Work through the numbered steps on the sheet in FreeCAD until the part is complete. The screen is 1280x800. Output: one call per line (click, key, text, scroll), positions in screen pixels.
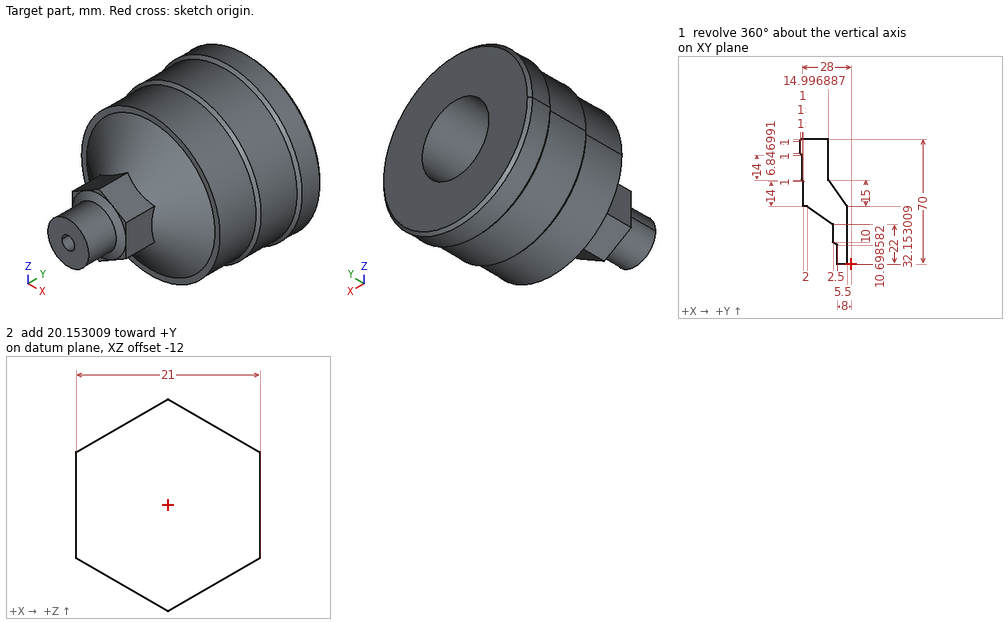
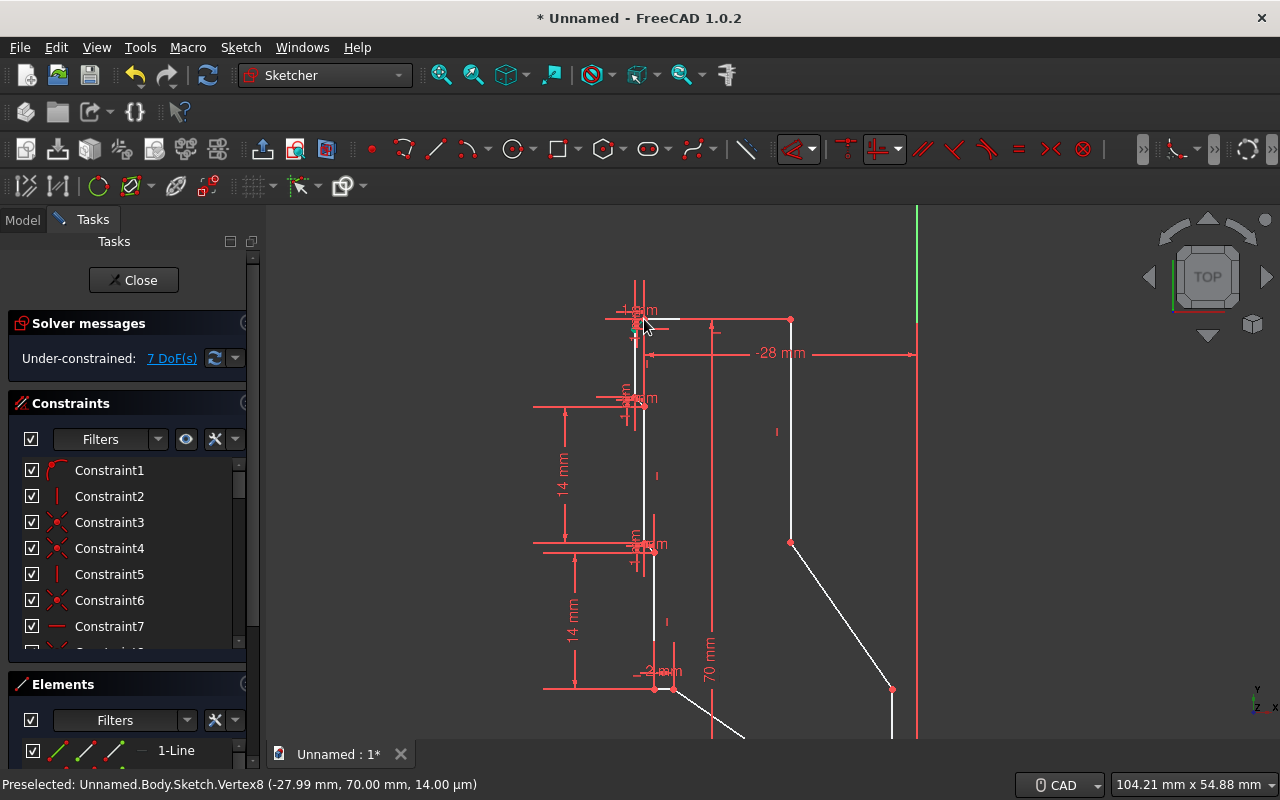
scroll(646, 319, down, 4)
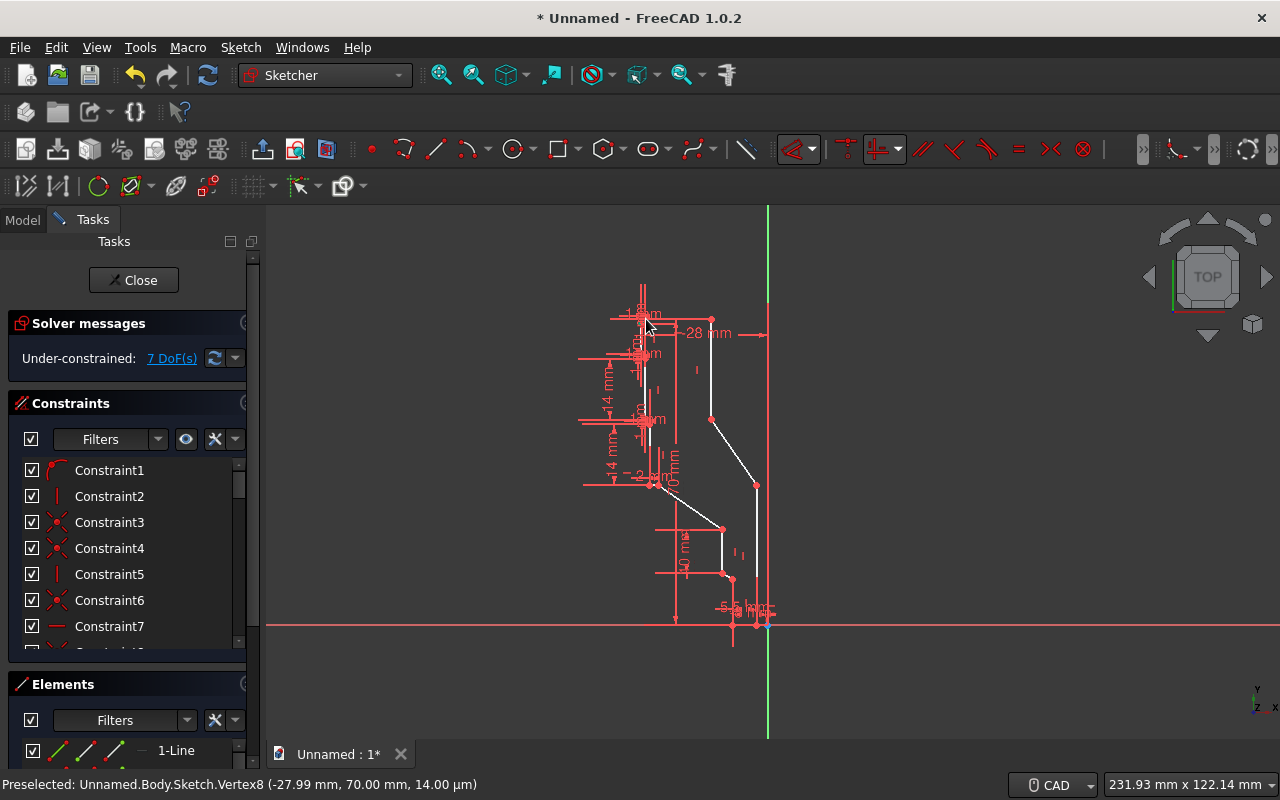
click(722, 530)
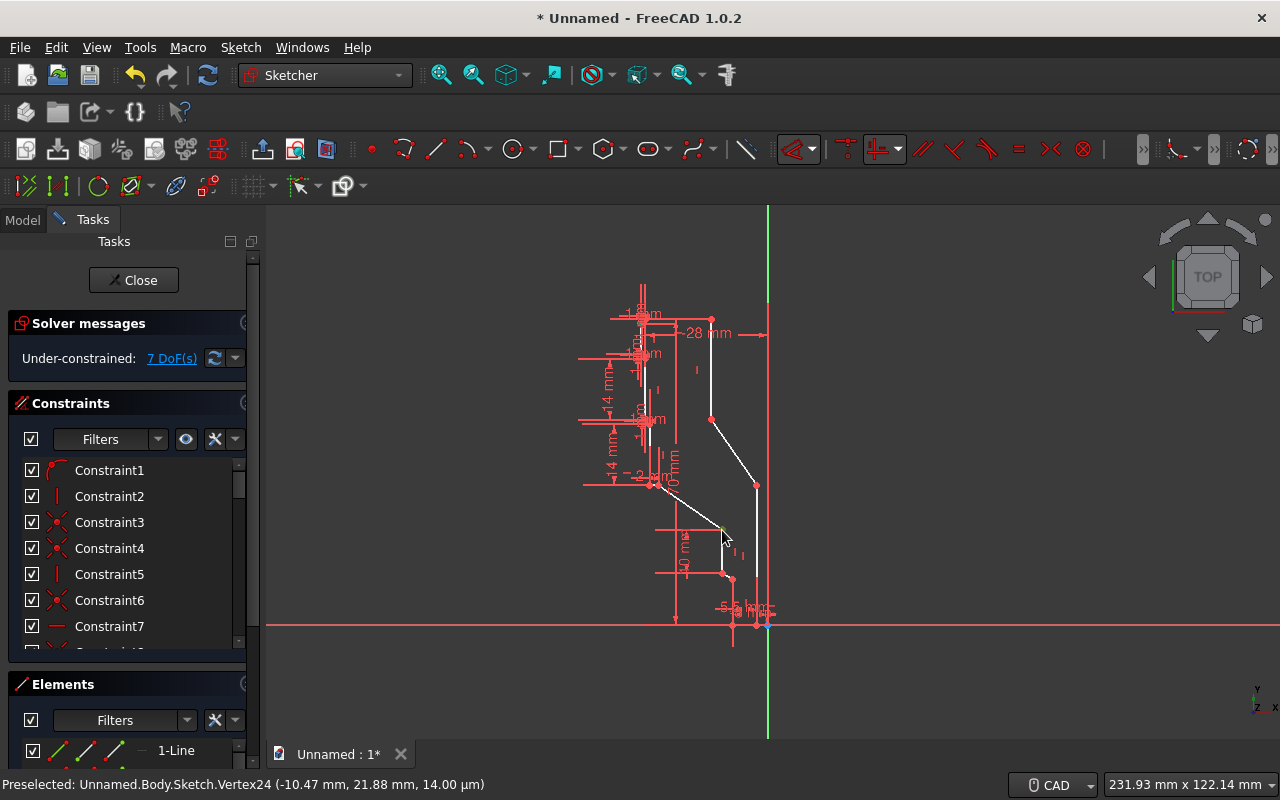
key(i)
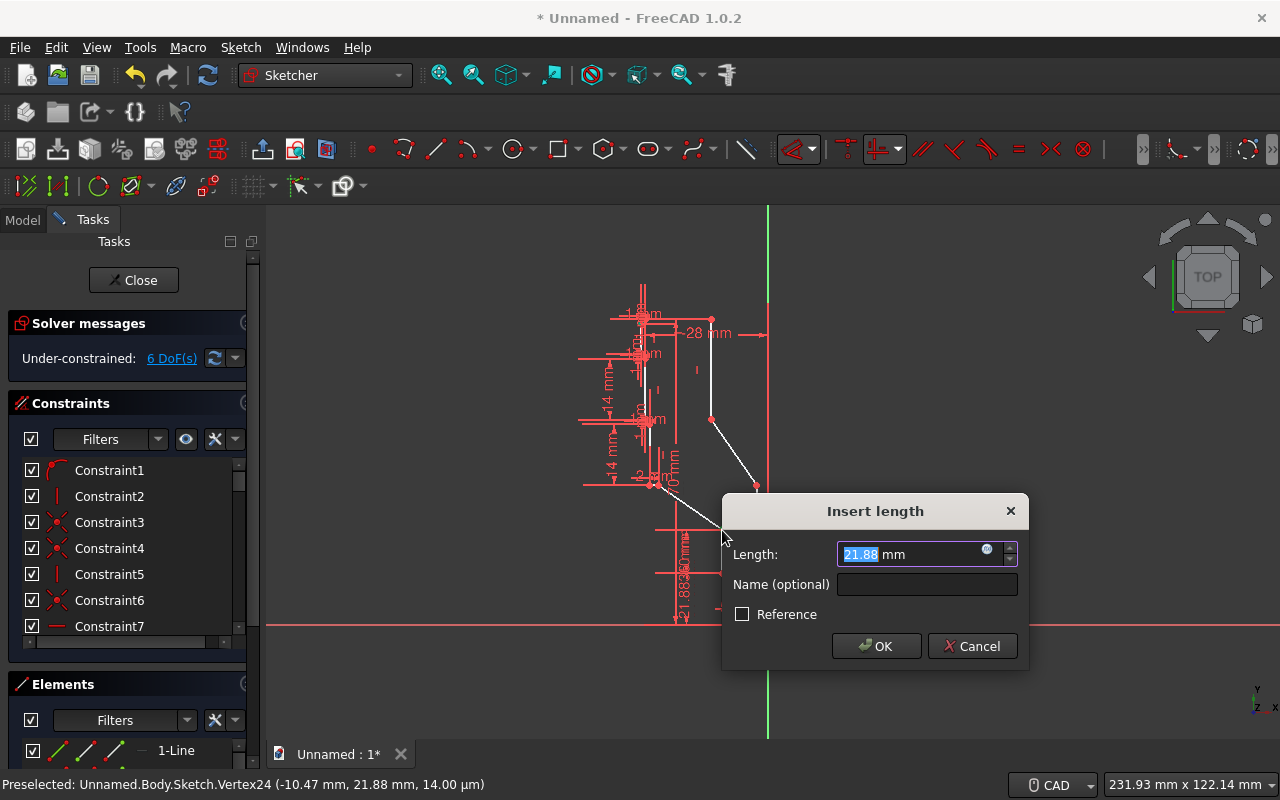
text(22)
key(Return)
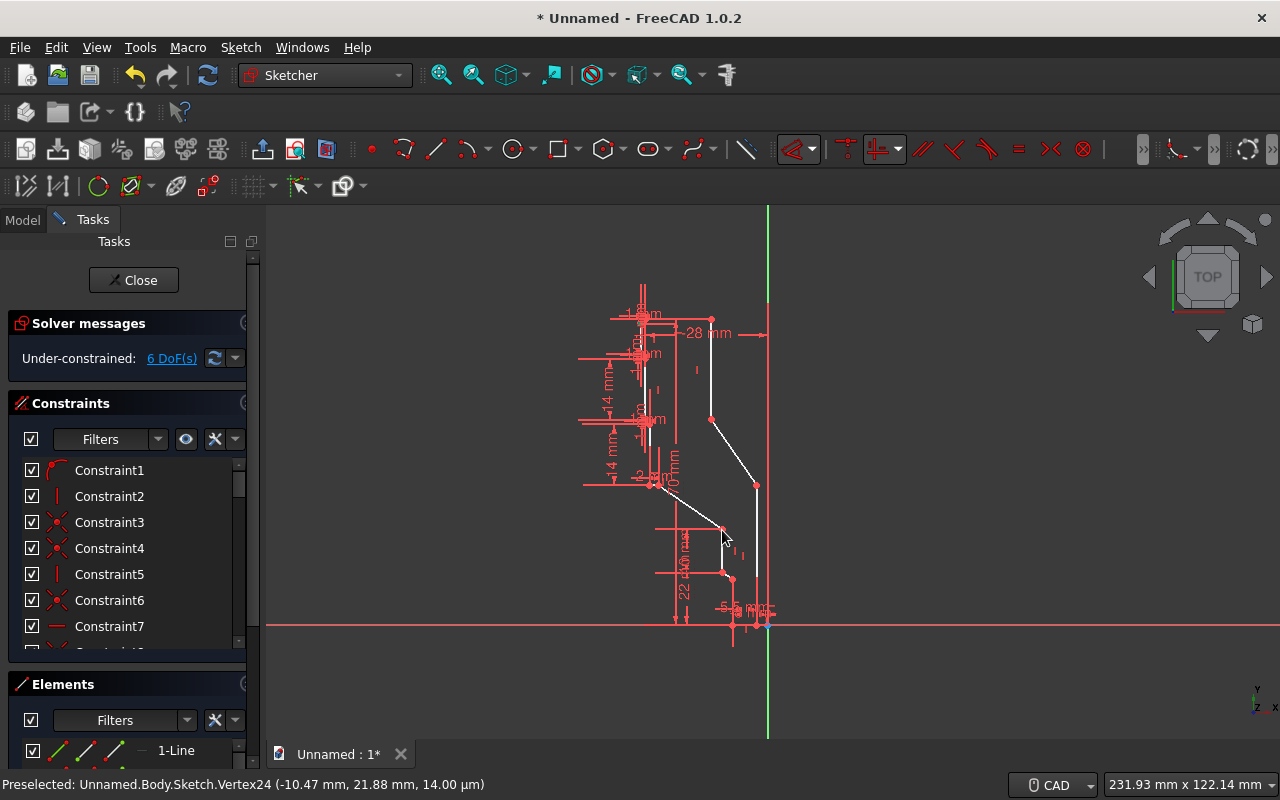
click(743, 466)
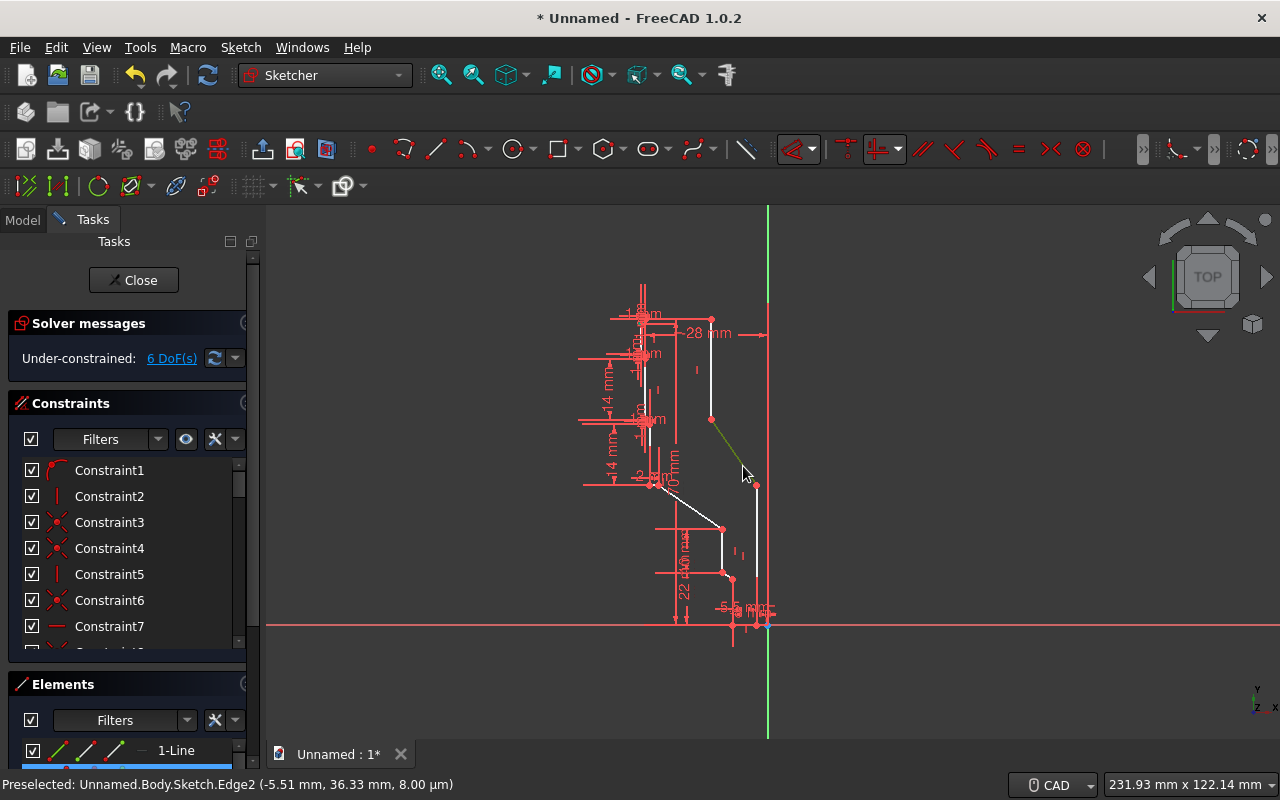
click(814, 150)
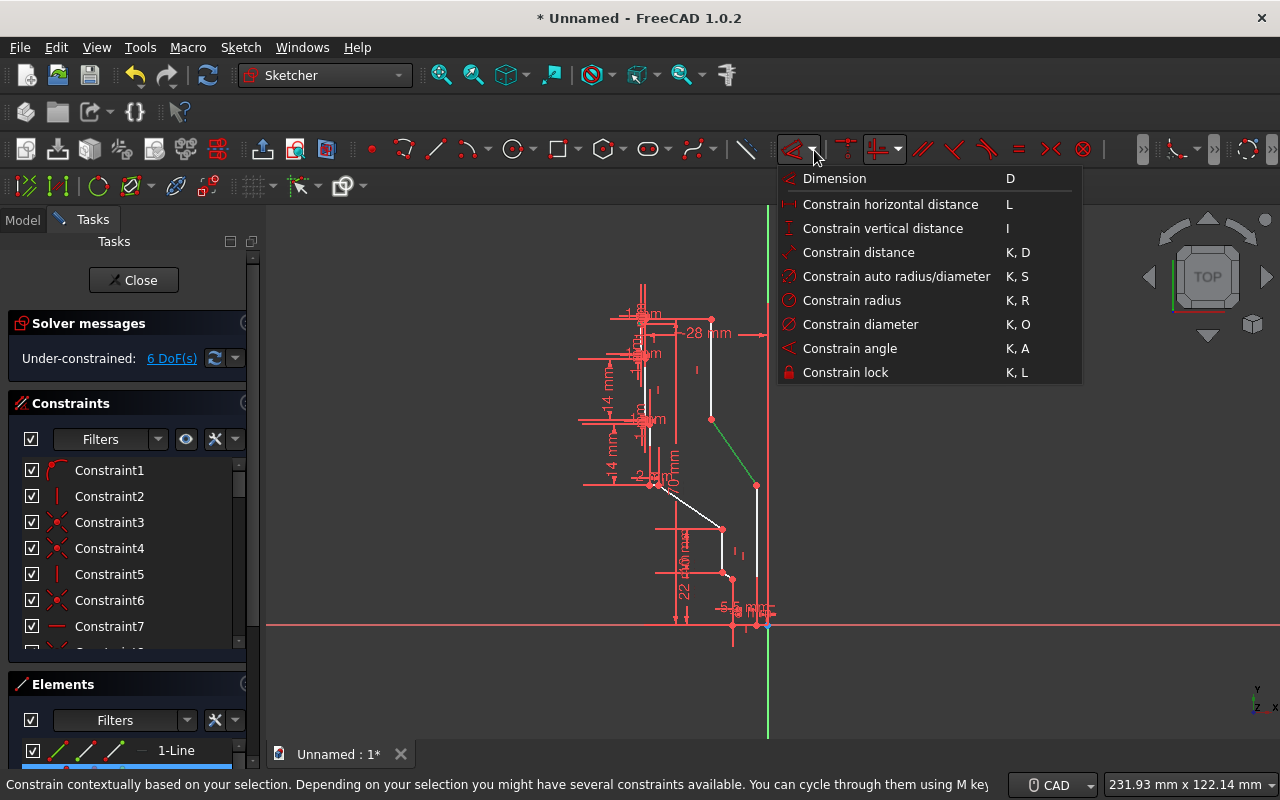
click(930, 228)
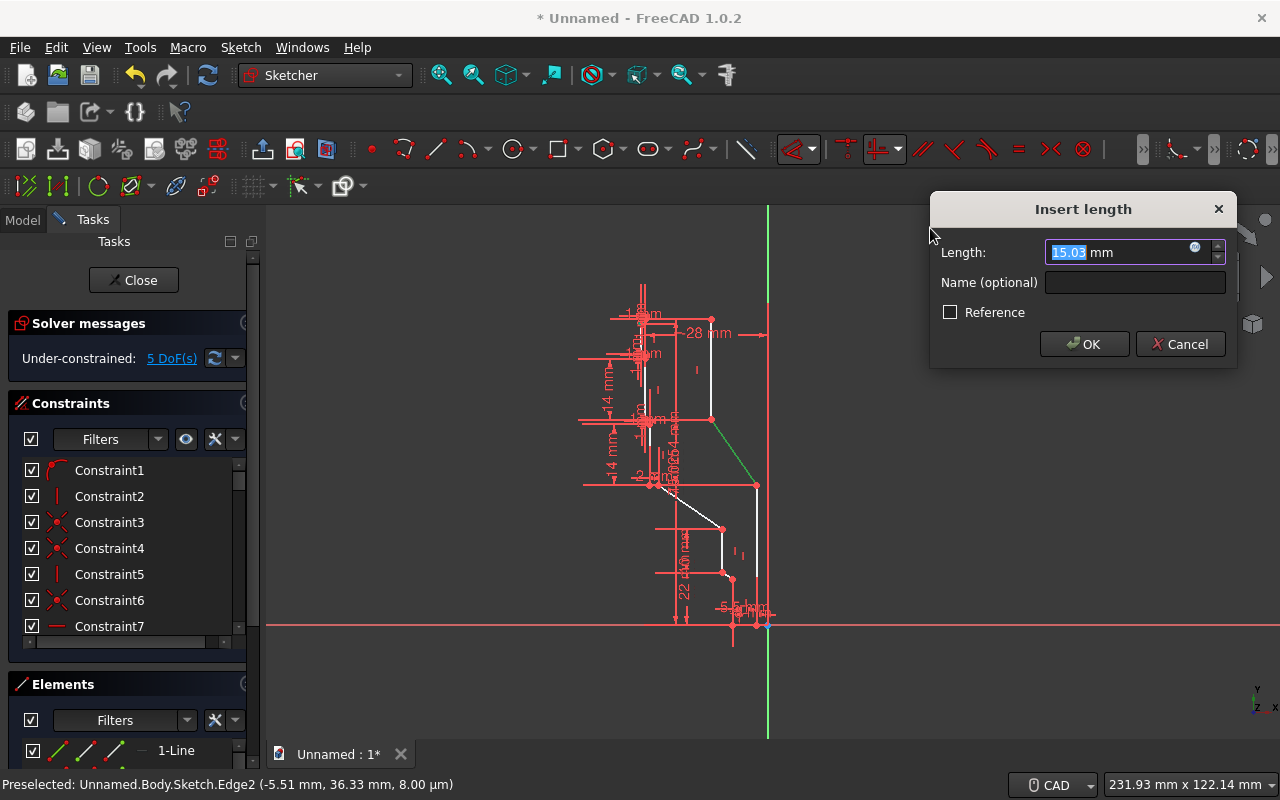
text(15)
key(Return)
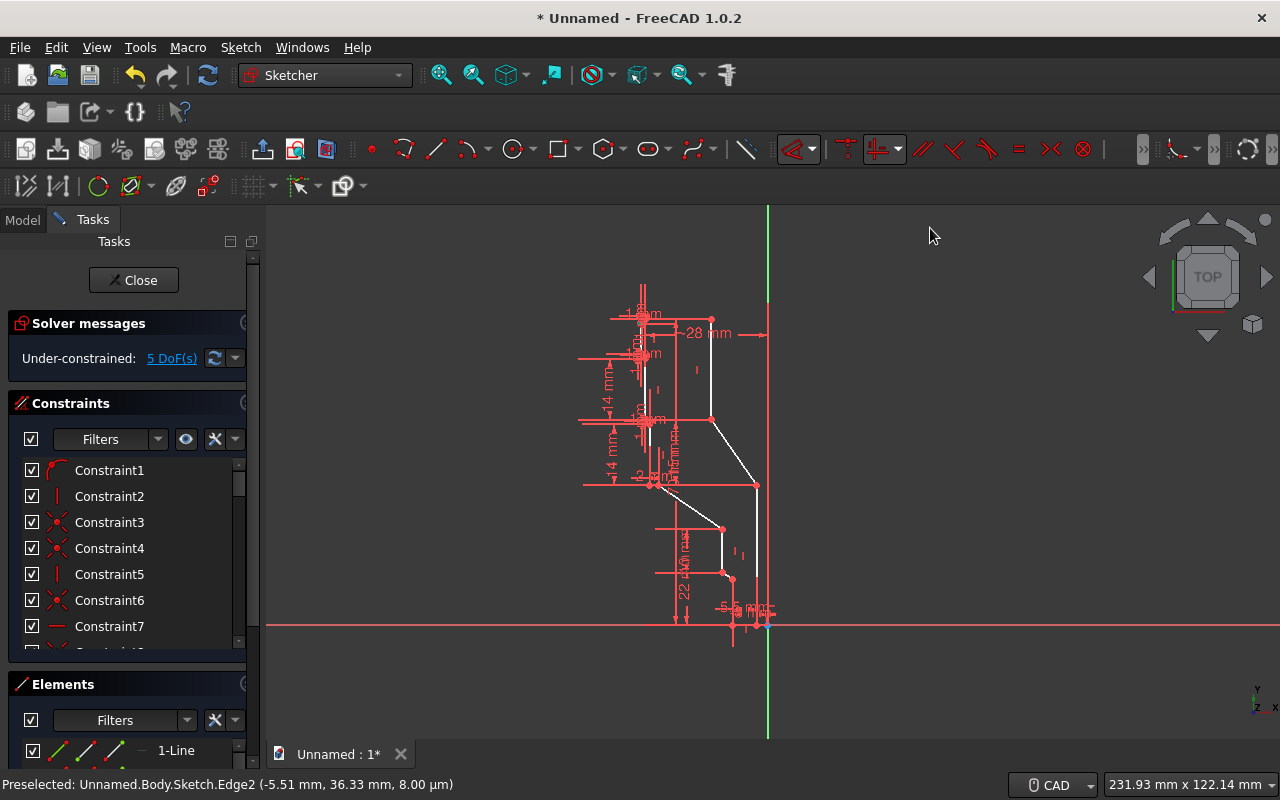
scroll(728, 576, up, 7)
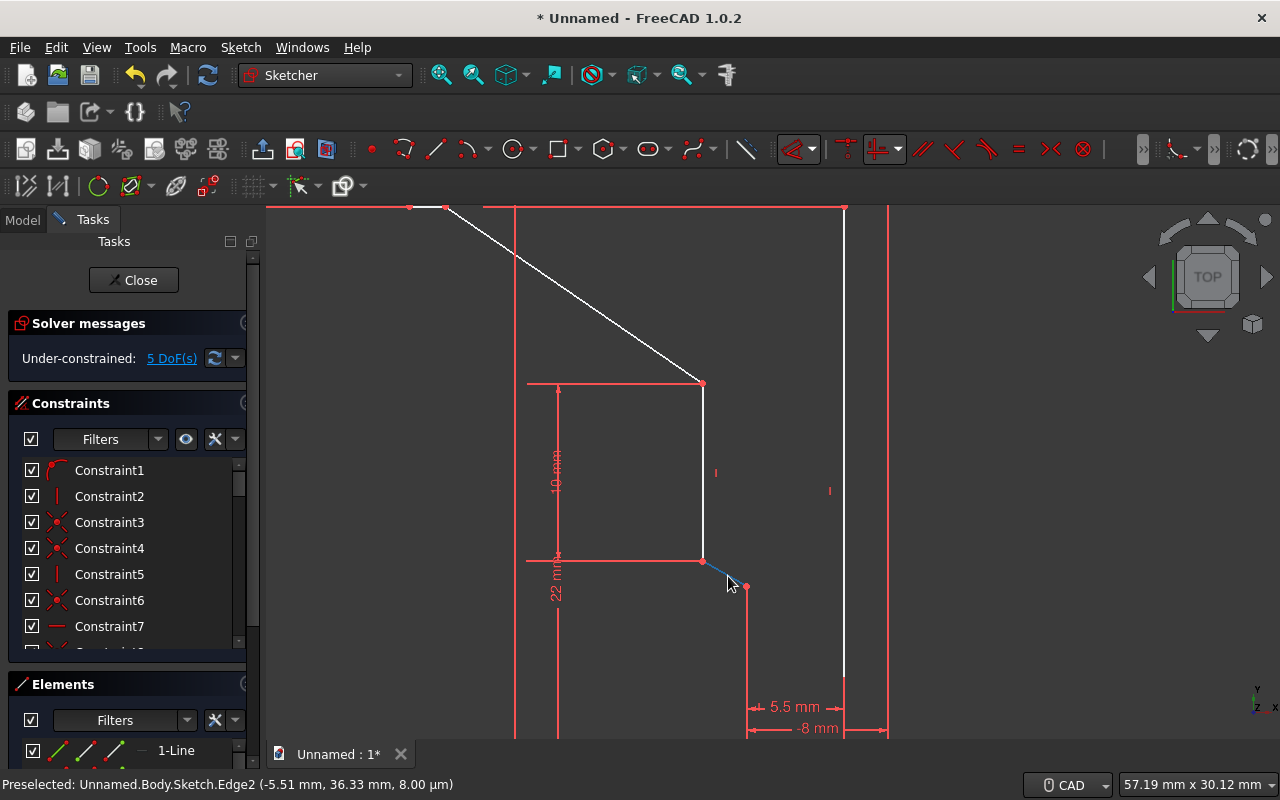
click(725, 574)